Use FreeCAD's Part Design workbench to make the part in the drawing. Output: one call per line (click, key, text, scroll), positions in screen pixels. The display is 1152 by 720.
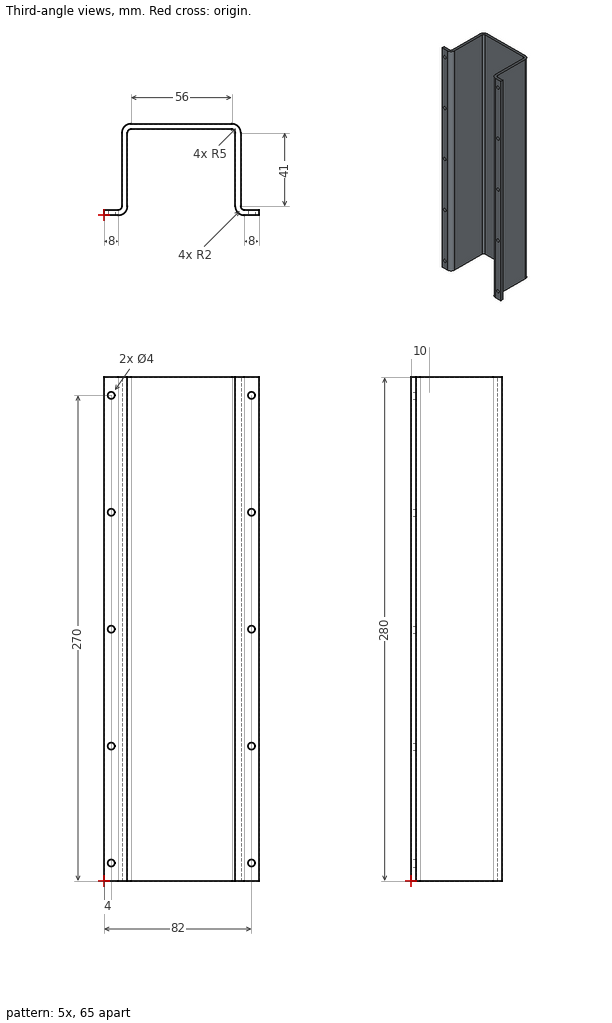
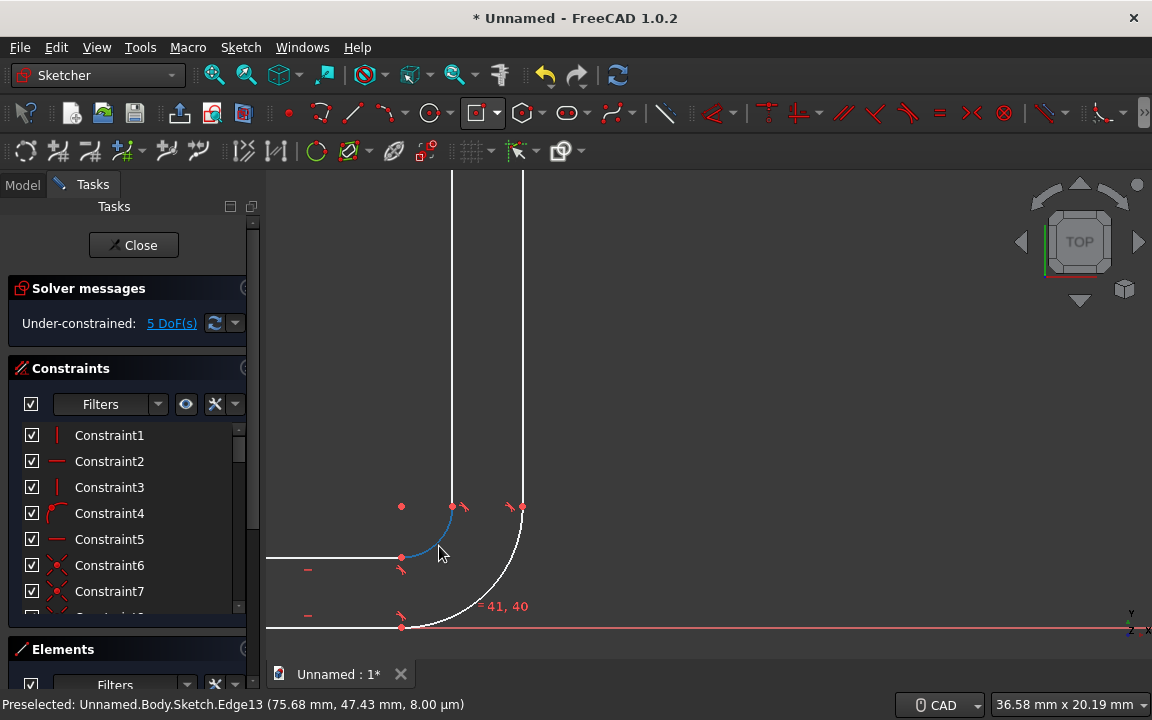
click(438, 543)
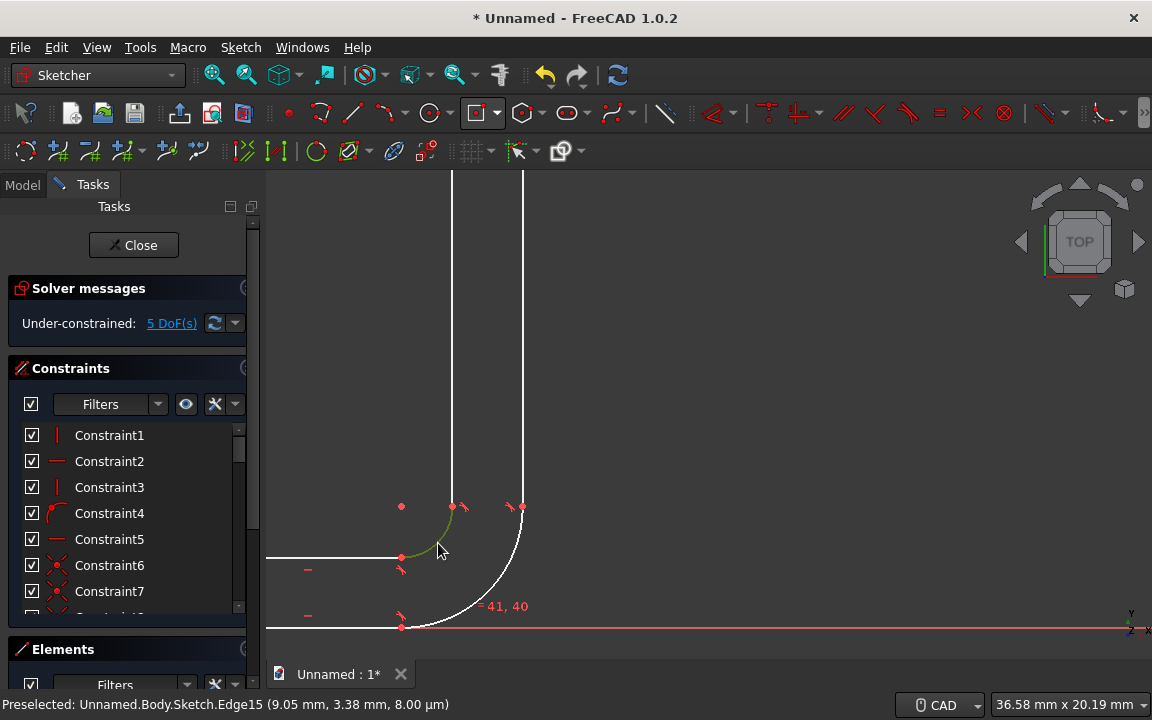
click(736, 114)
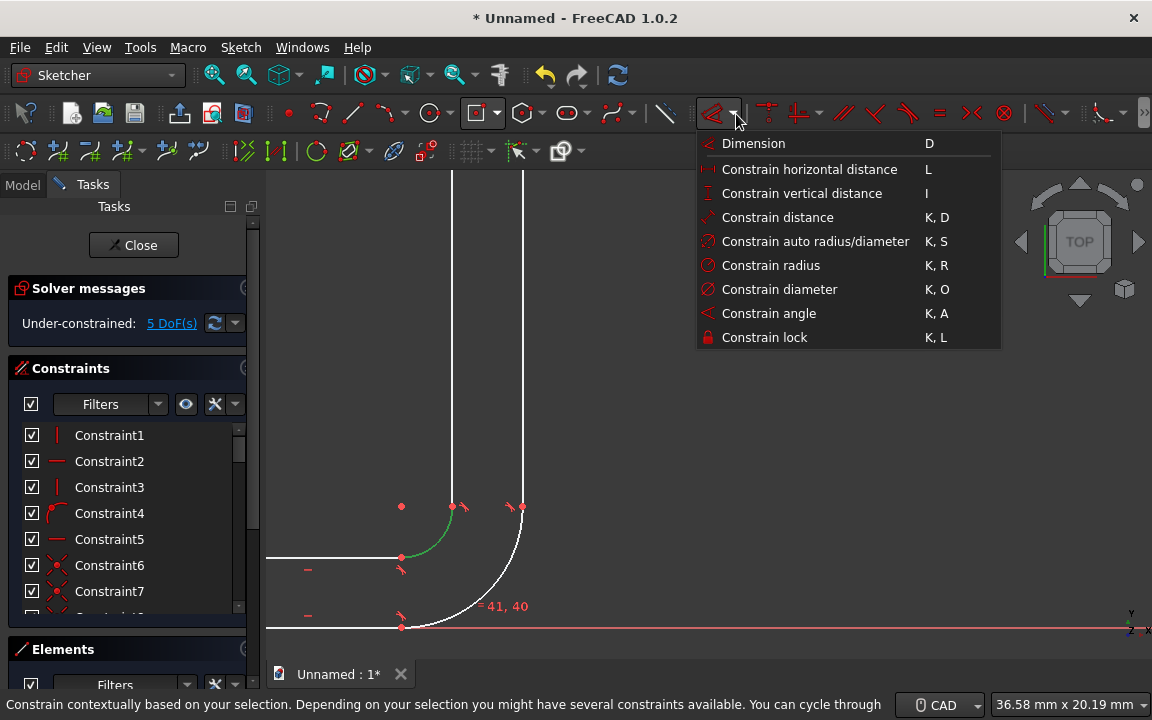
click(849, 265)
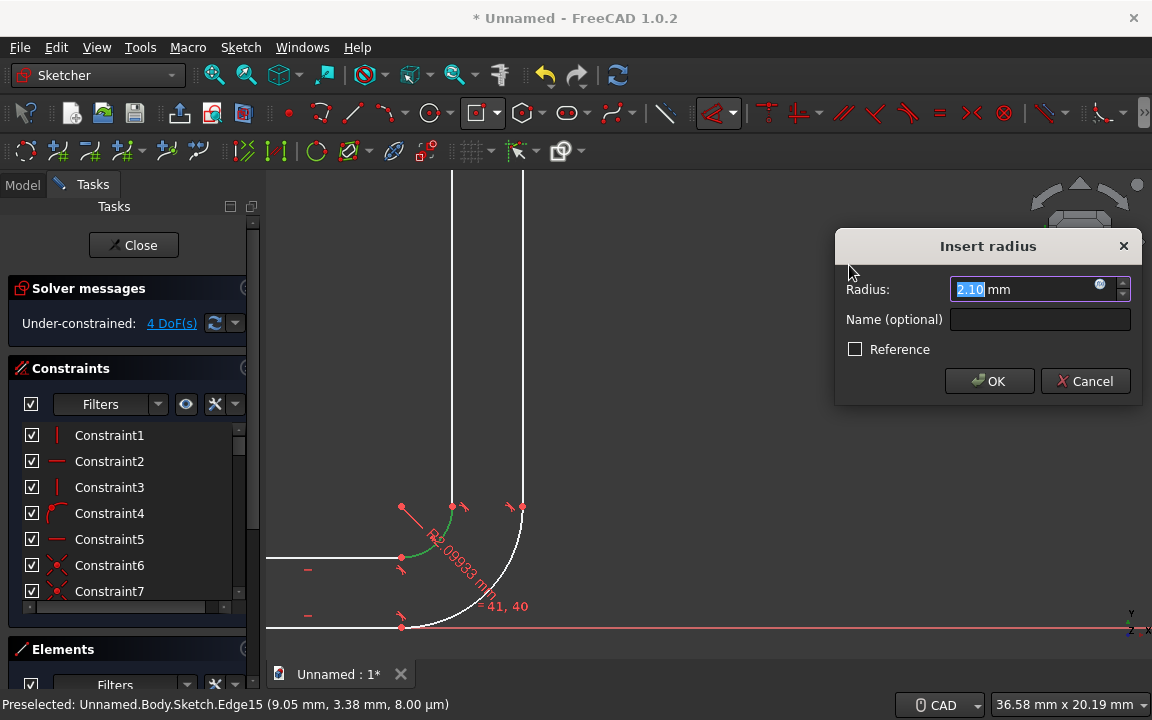
text(2)
key(Return)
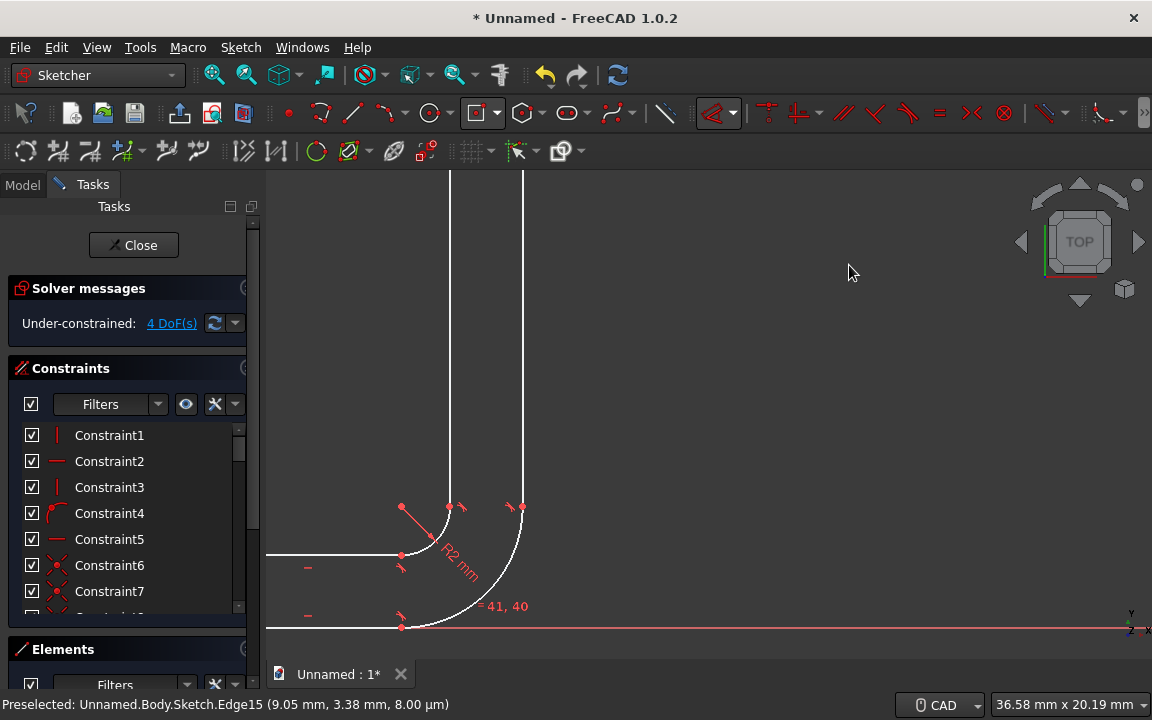
scroll(439, 547, down, 7)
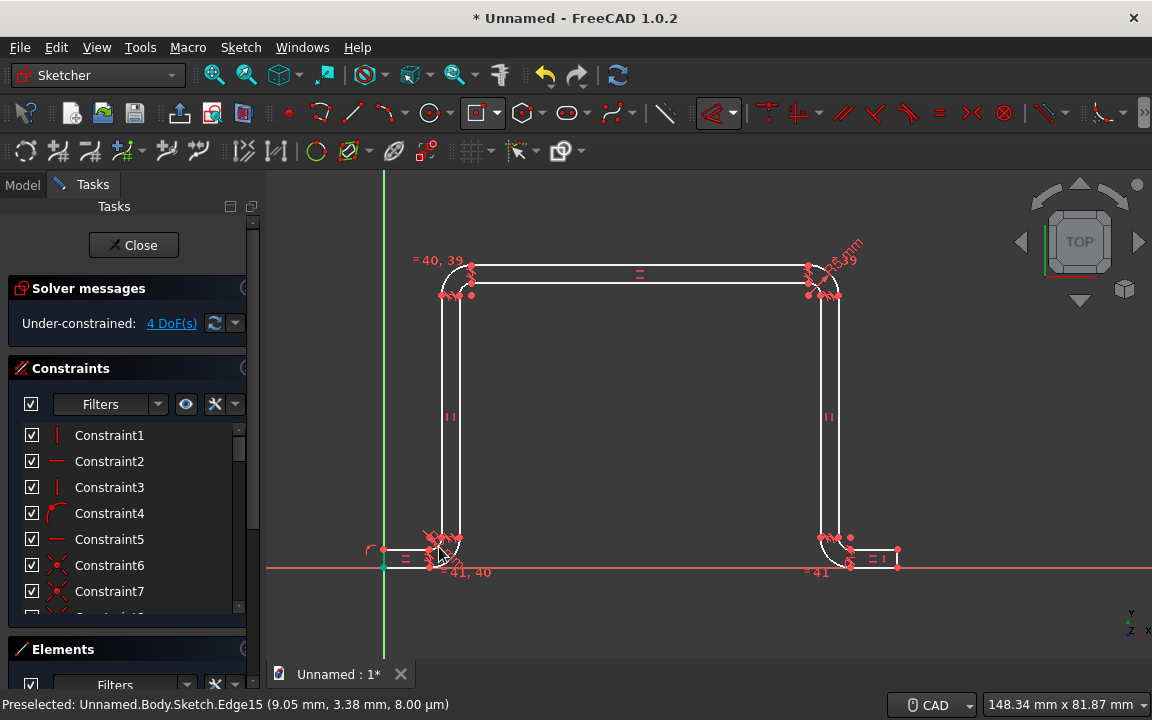
click(416, 550)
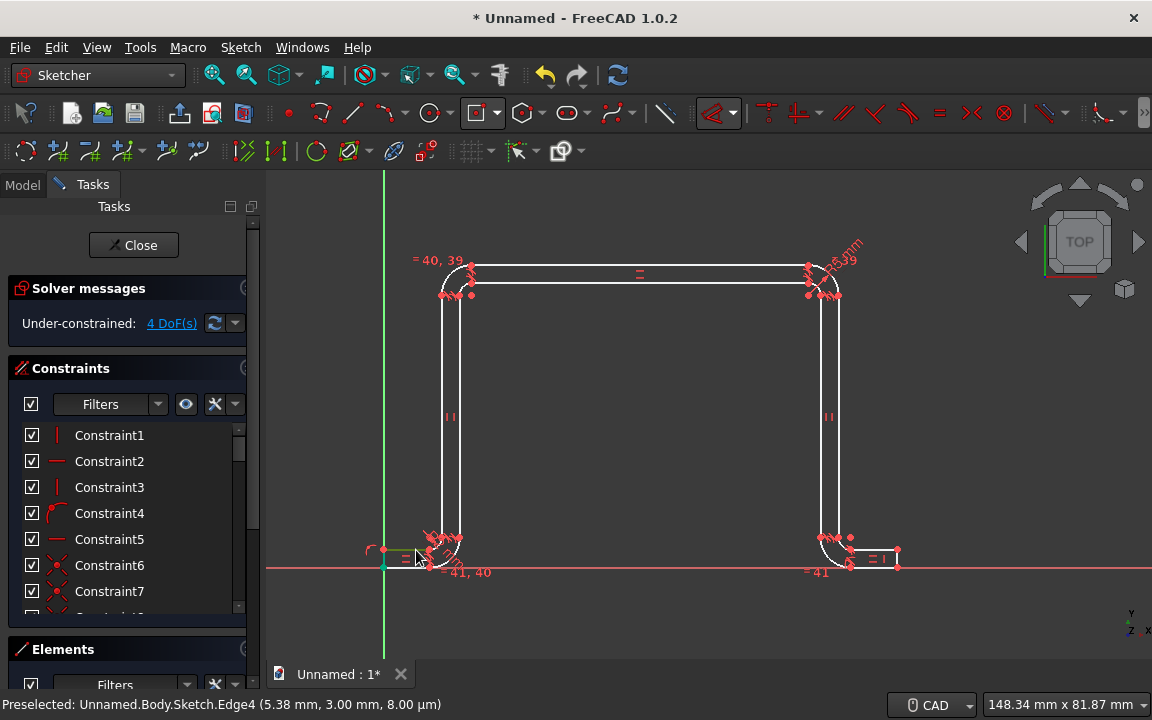
key(l)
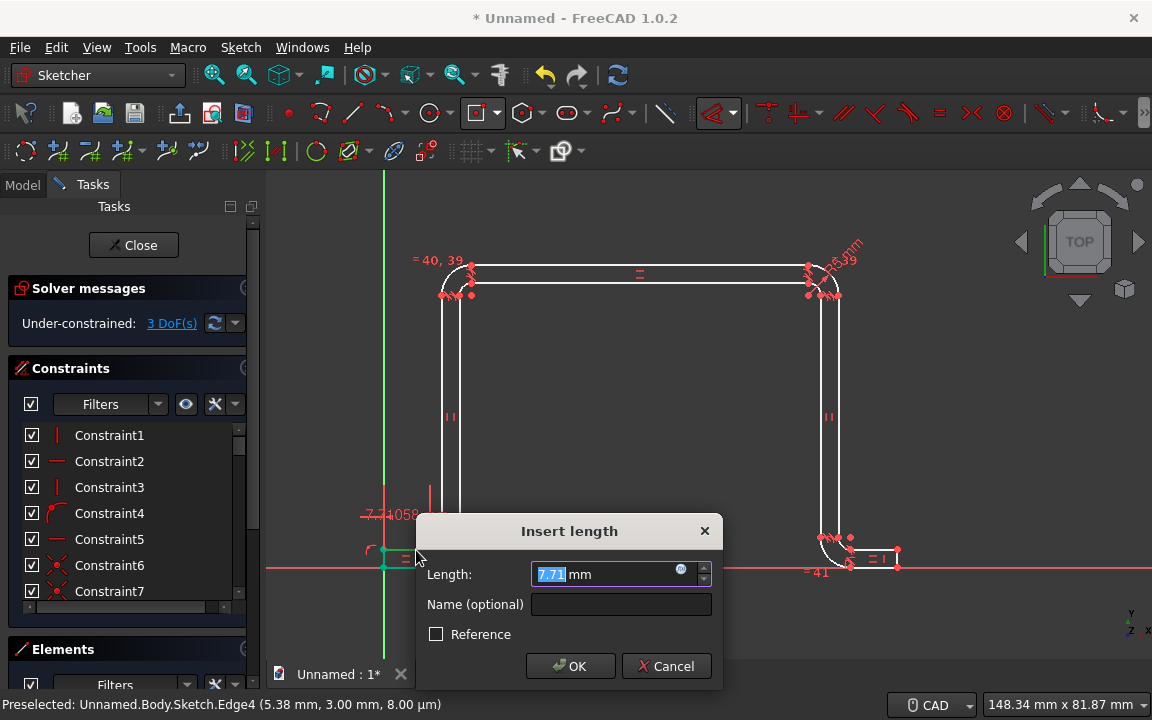
text(8)
key(Return)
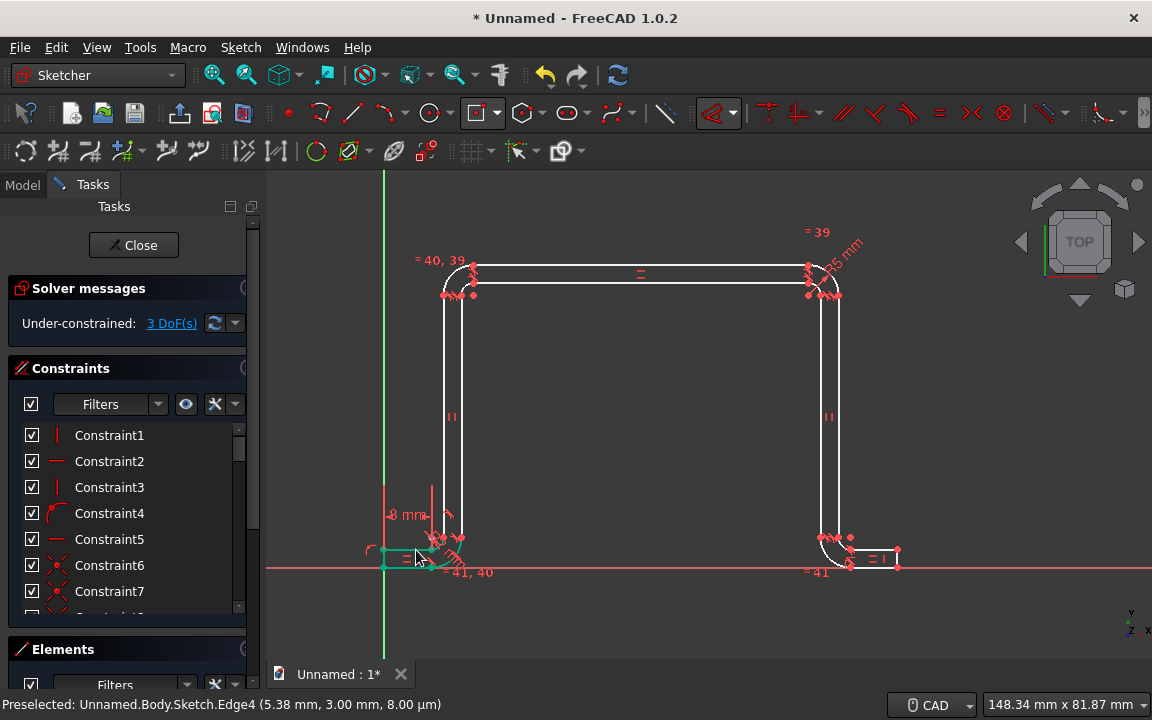
click(865, 568)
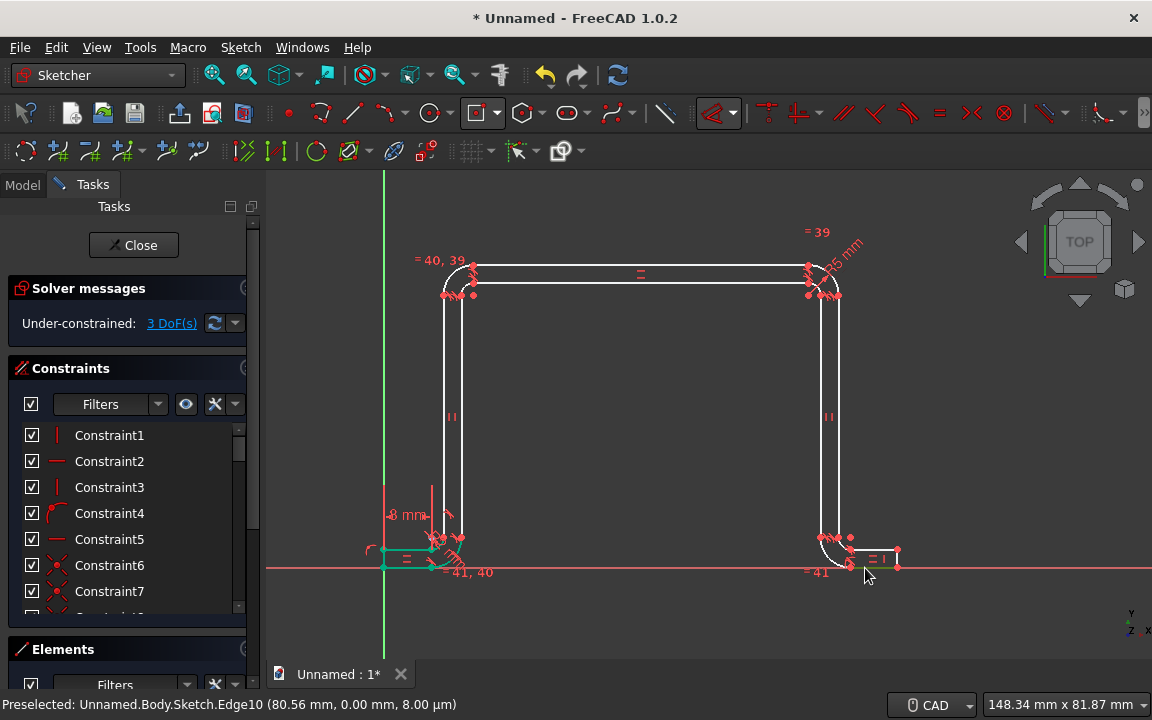
click(736, 114)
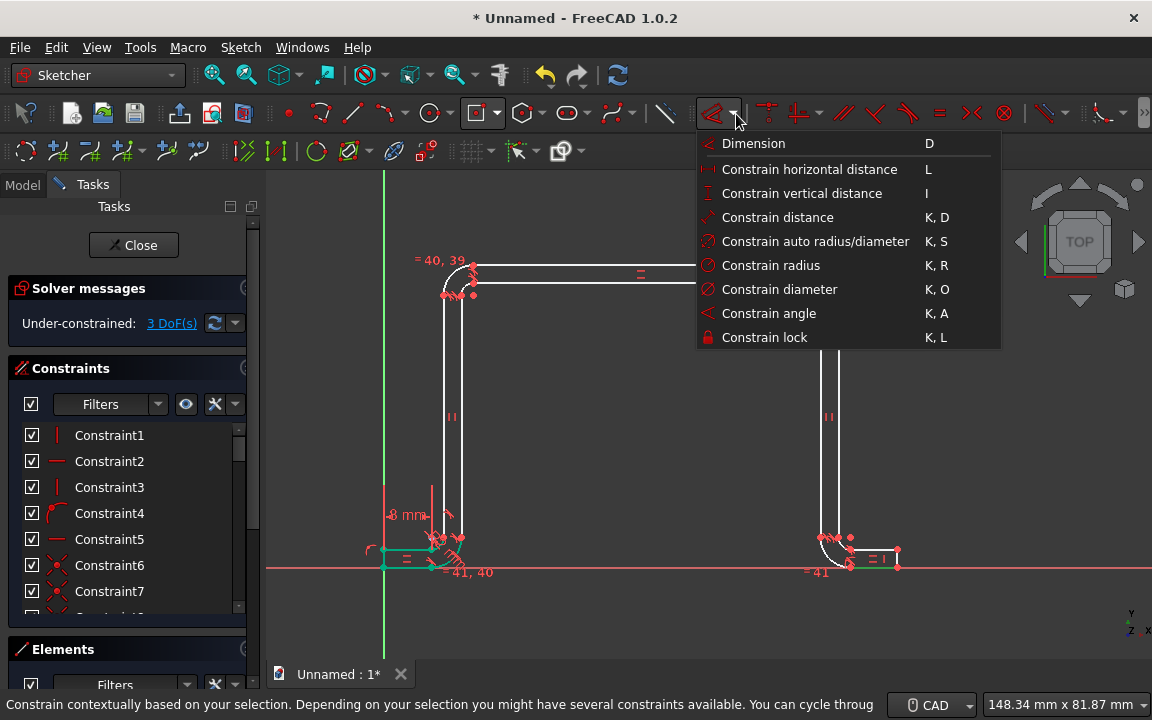
click(849, 169)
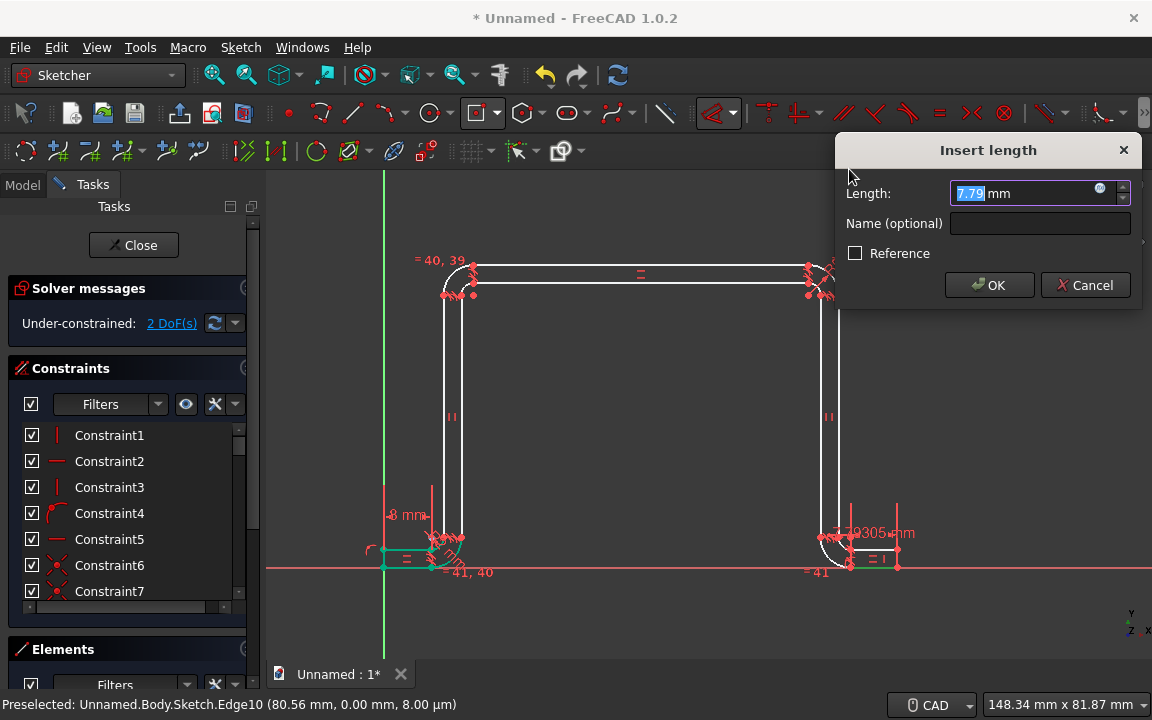
text(8)
key(Return)